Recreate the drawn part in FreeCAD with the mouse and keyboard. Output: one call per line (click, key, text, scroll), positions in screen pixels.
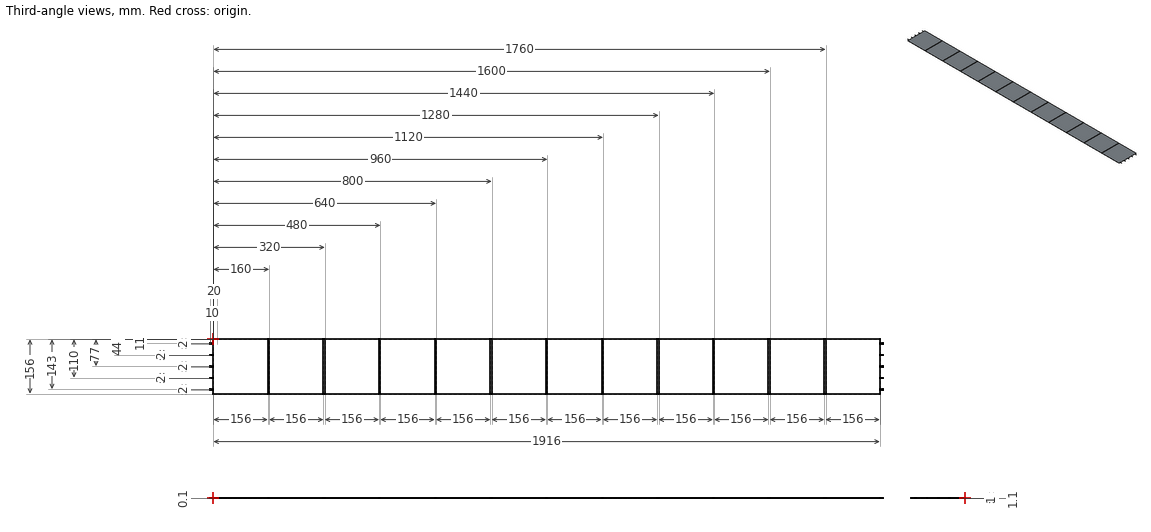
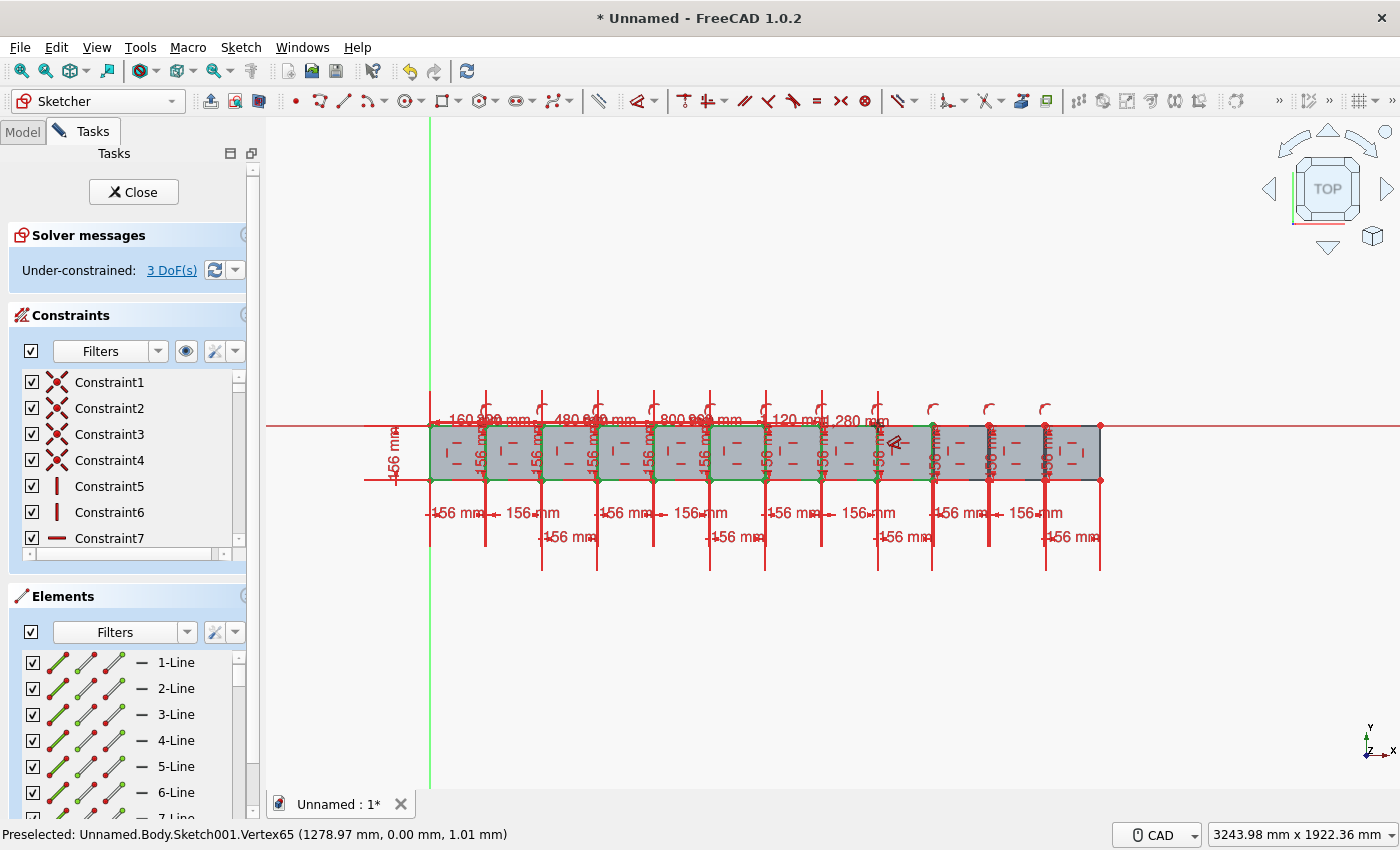
scroll(934, 426, up, 13)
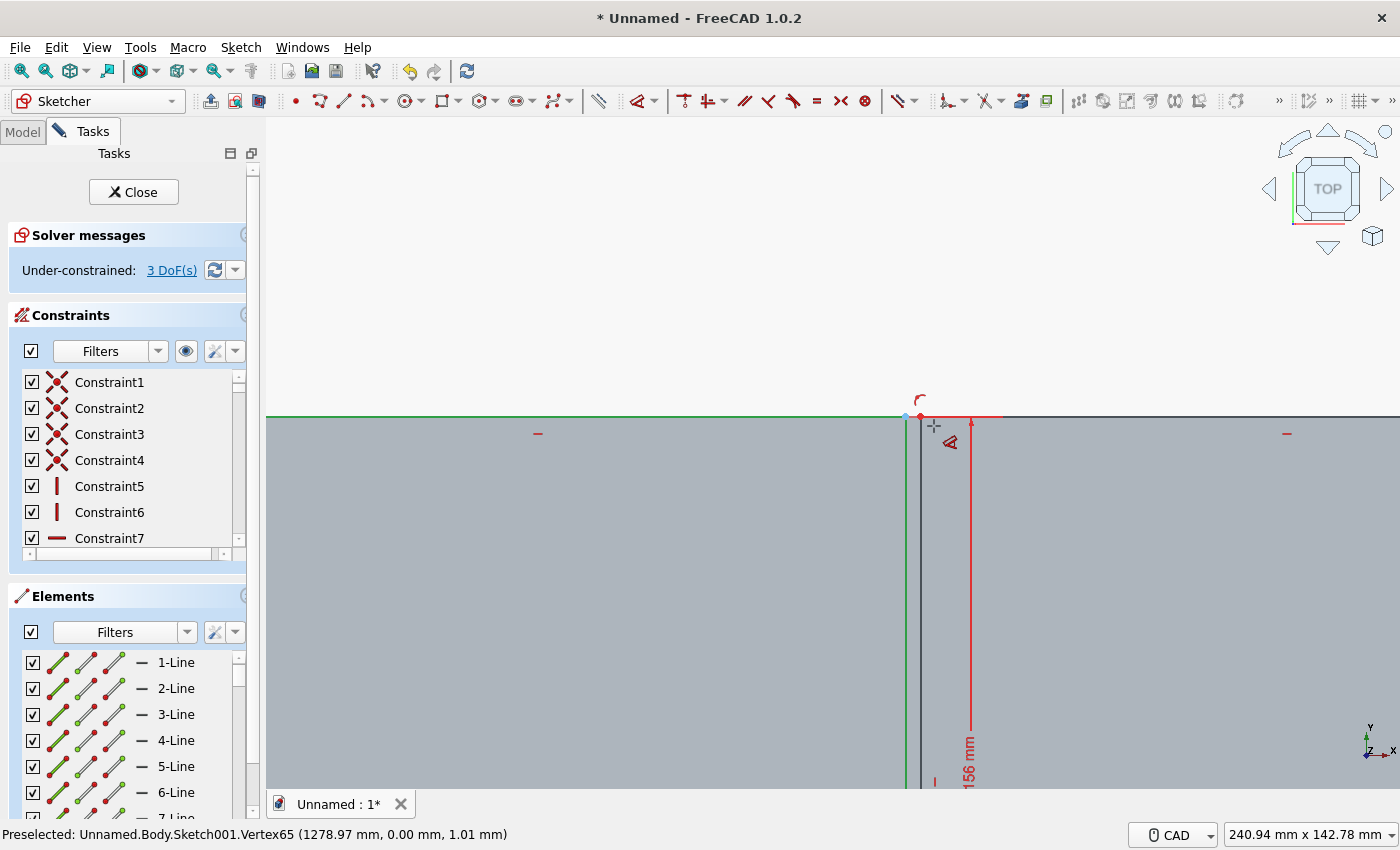
click(921, 417)
click(607, 383)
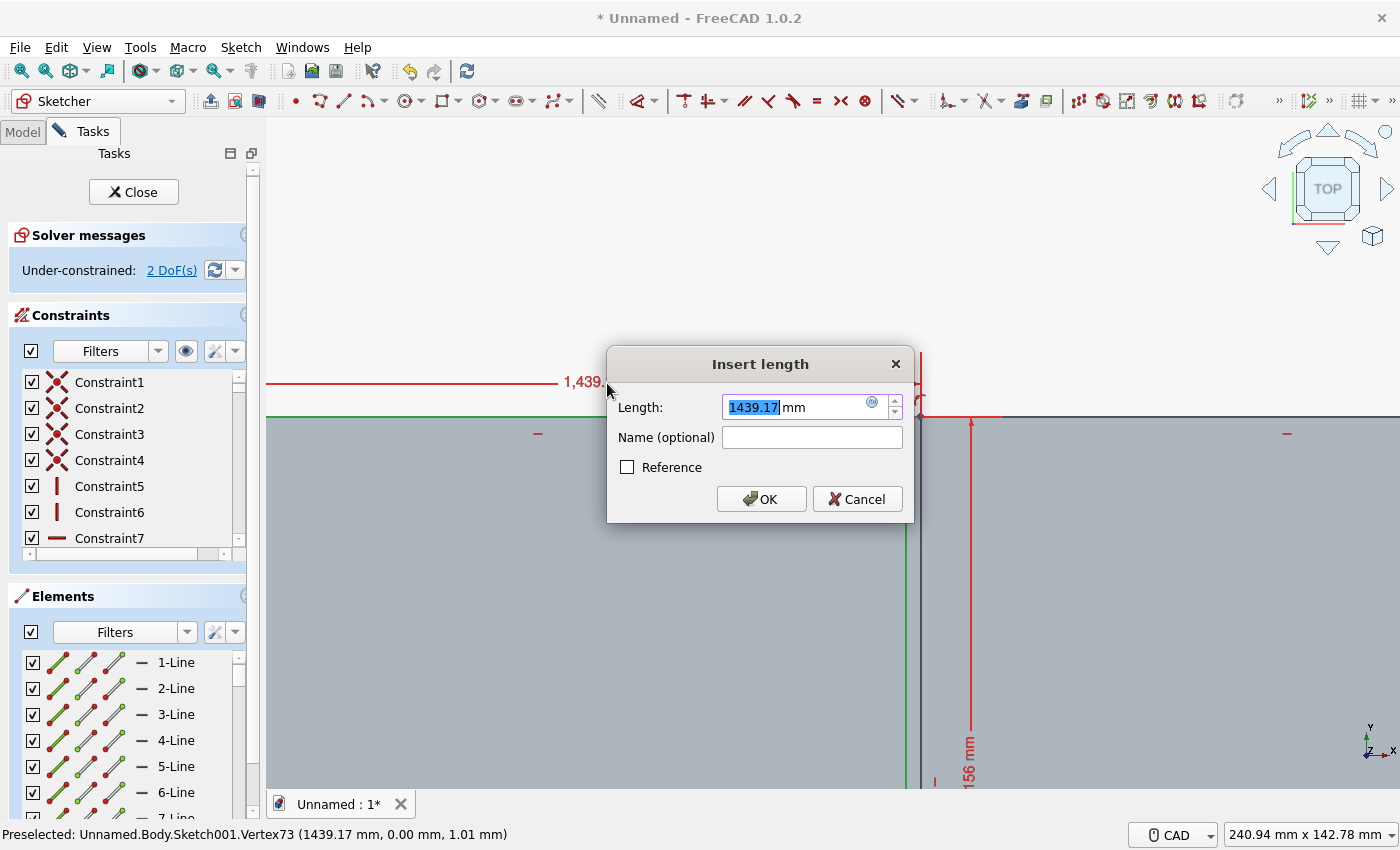
text(1440)
key(Return)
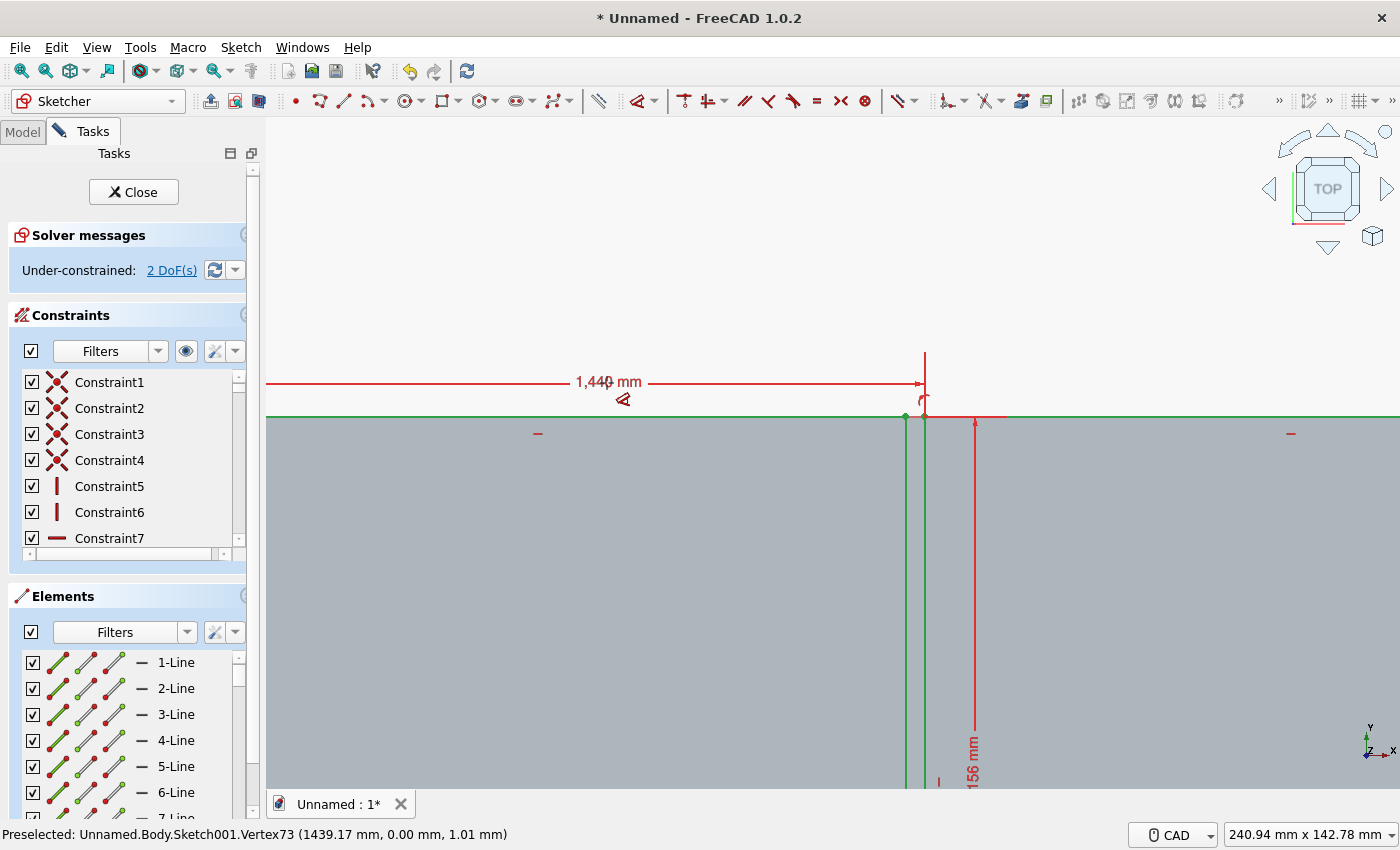
scroll(934, 426, down, 13)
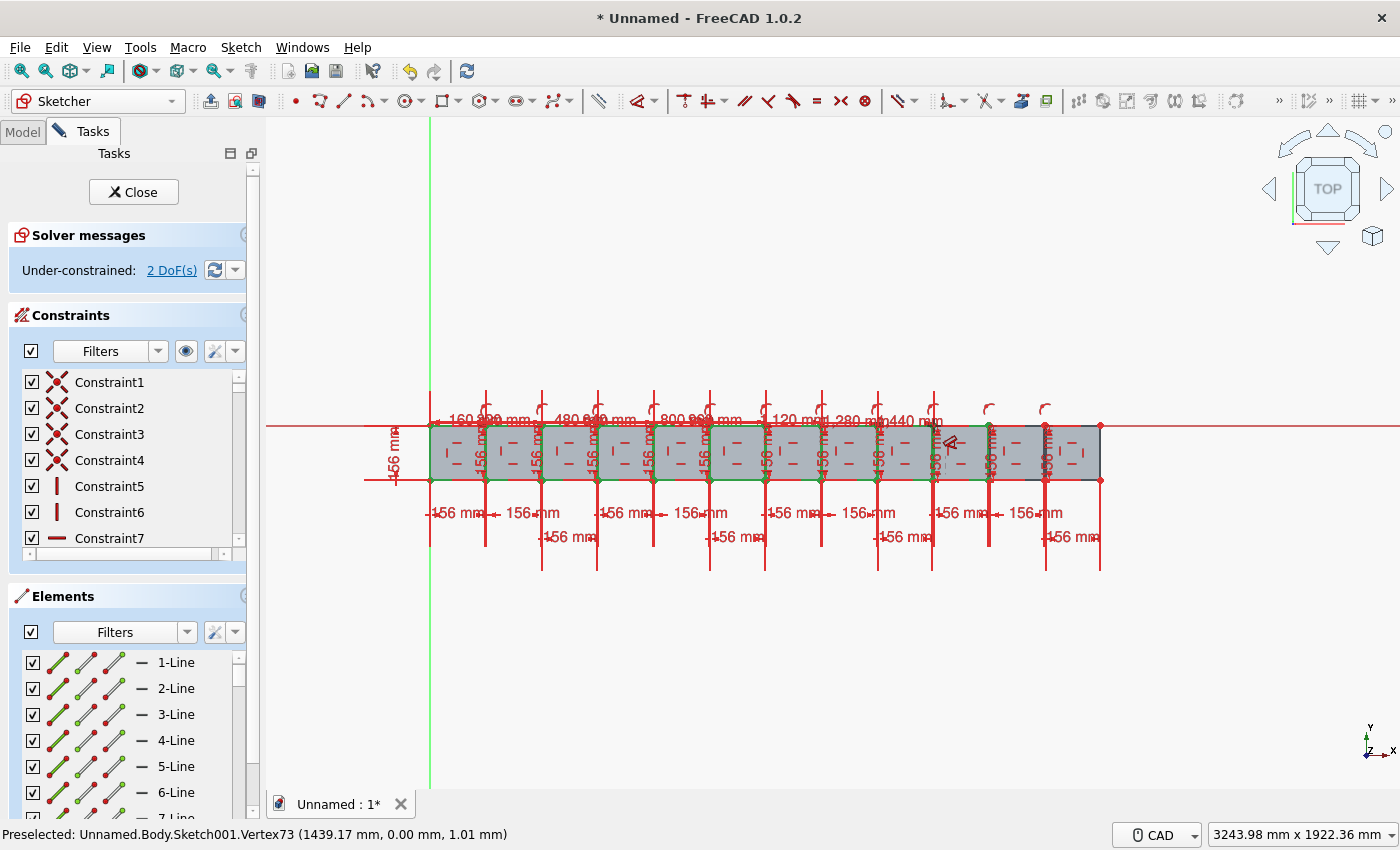
scroll(990, 426, up, 12)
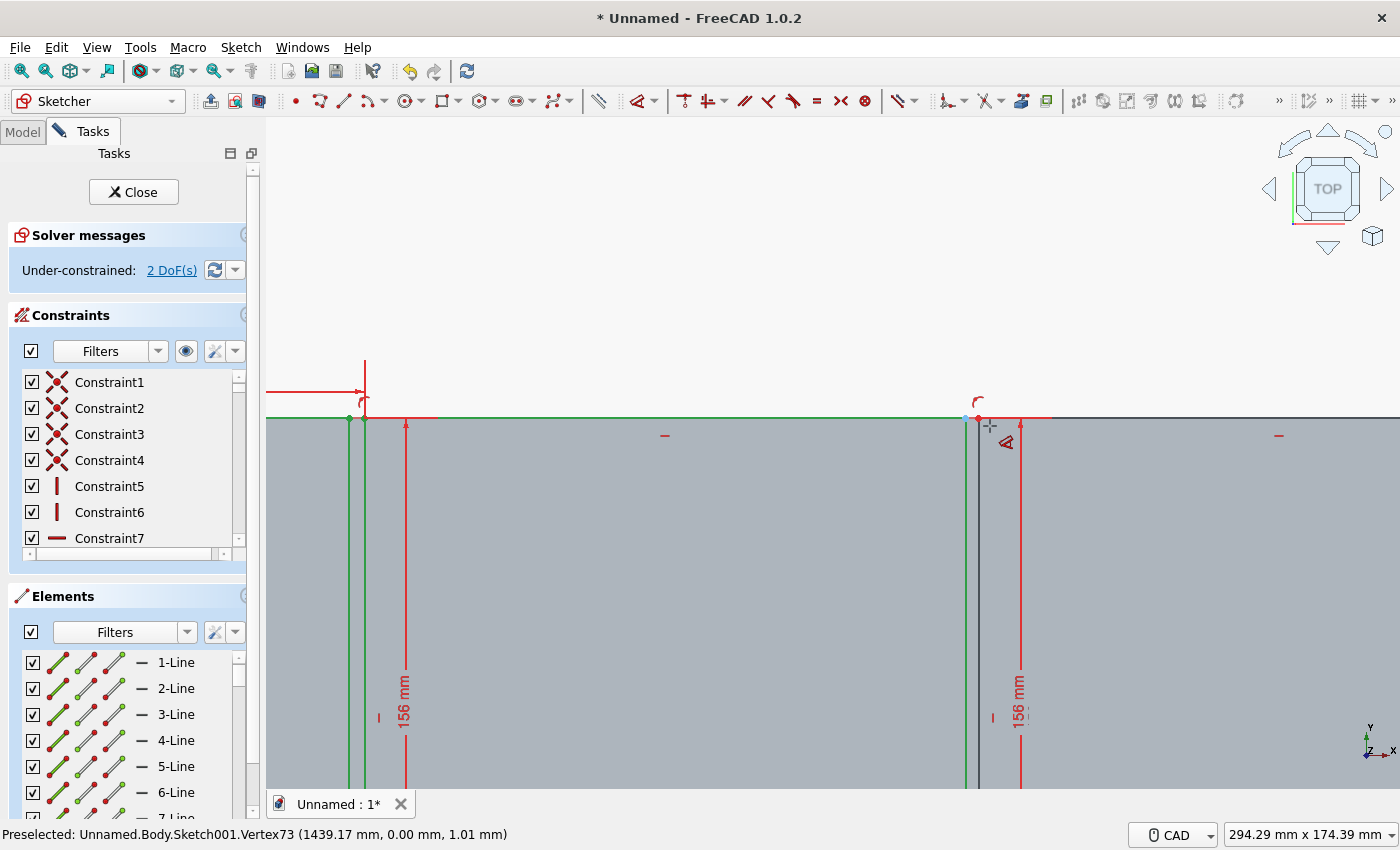
click(979, 418)
click(636, 384)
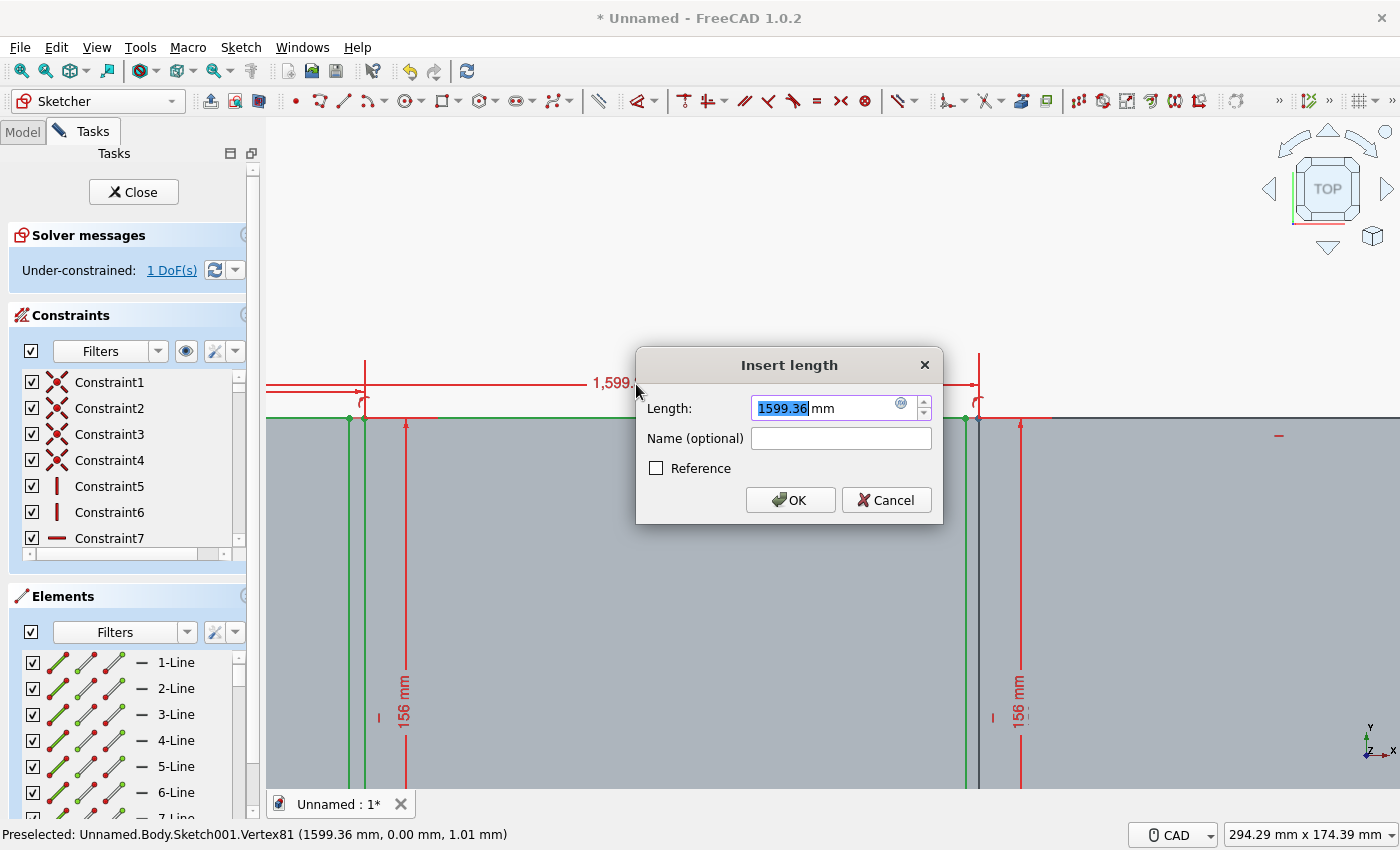
text(1600)
key(Return)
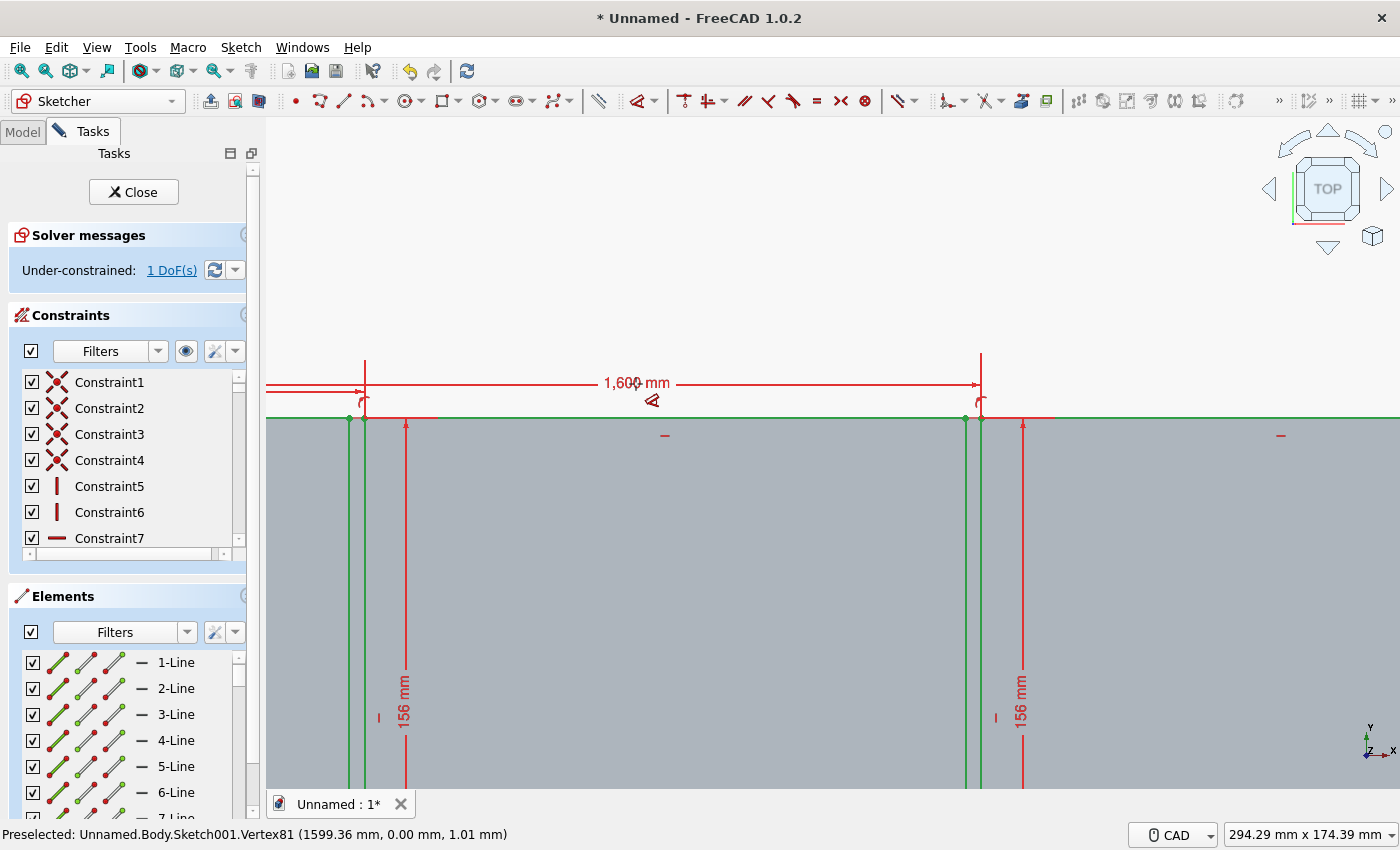
scroll(990, 426, down, 12)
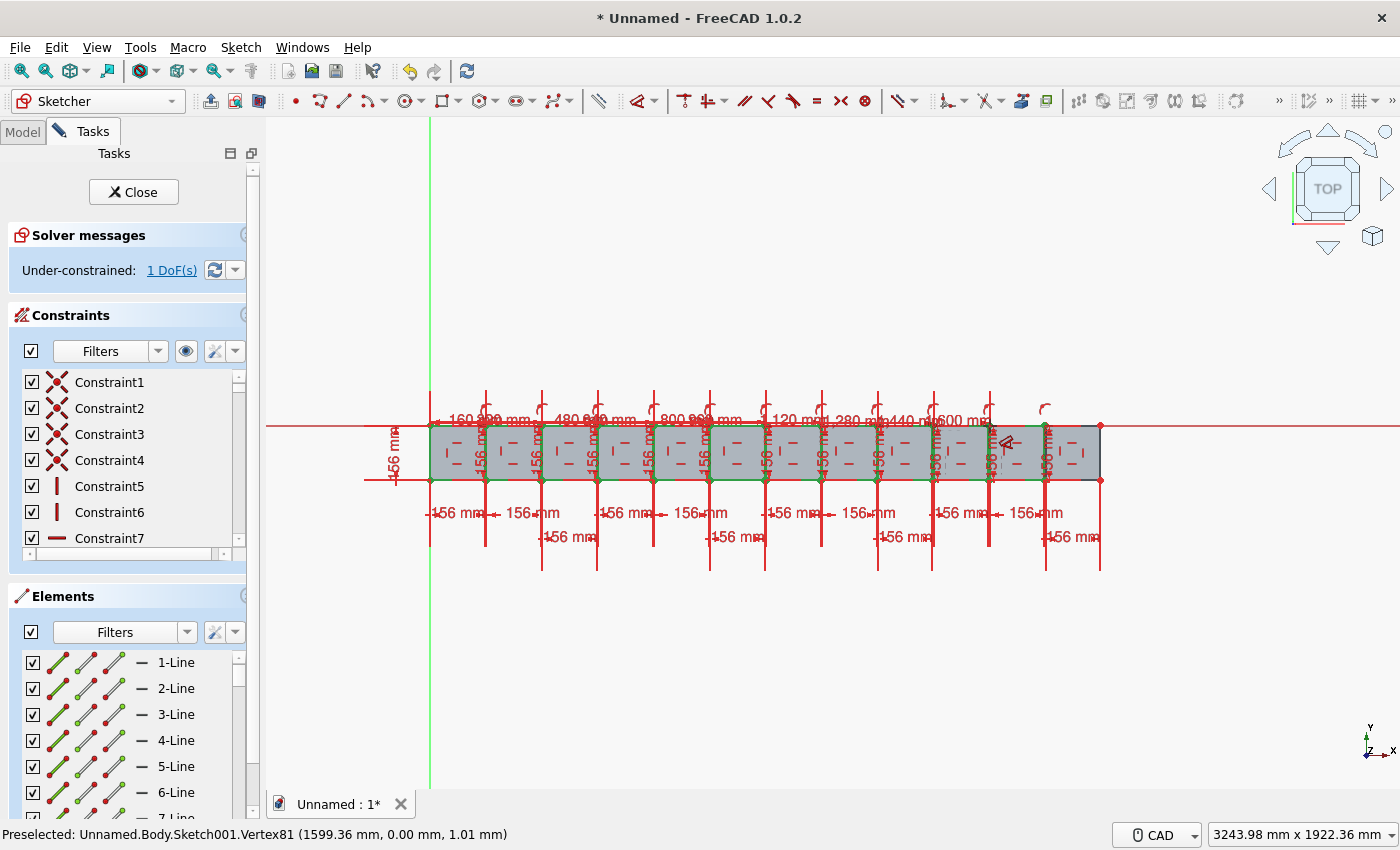
scroll(1046, 426, up, 12)